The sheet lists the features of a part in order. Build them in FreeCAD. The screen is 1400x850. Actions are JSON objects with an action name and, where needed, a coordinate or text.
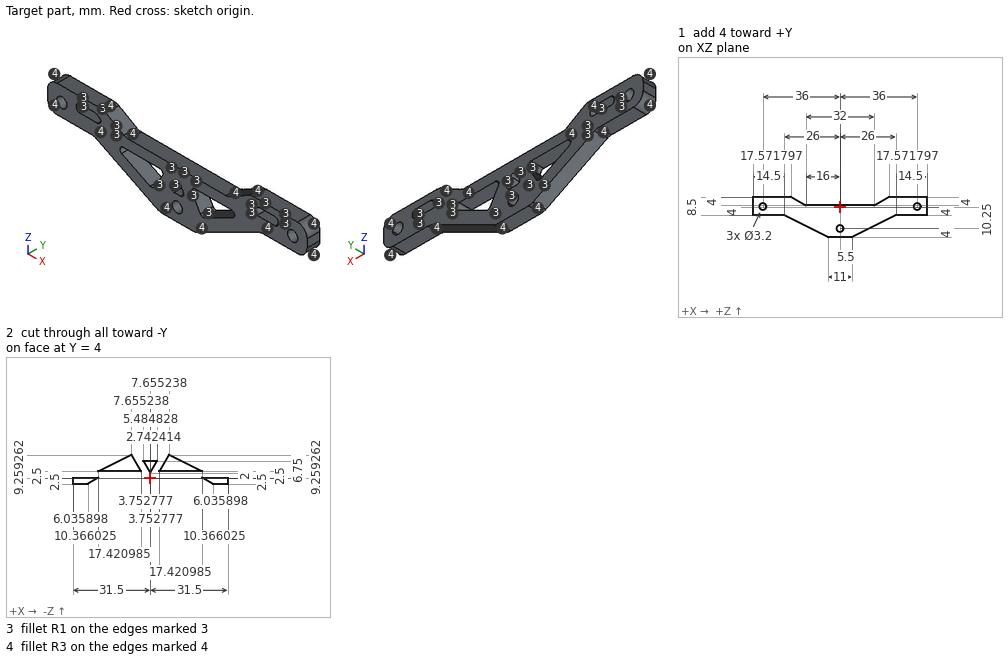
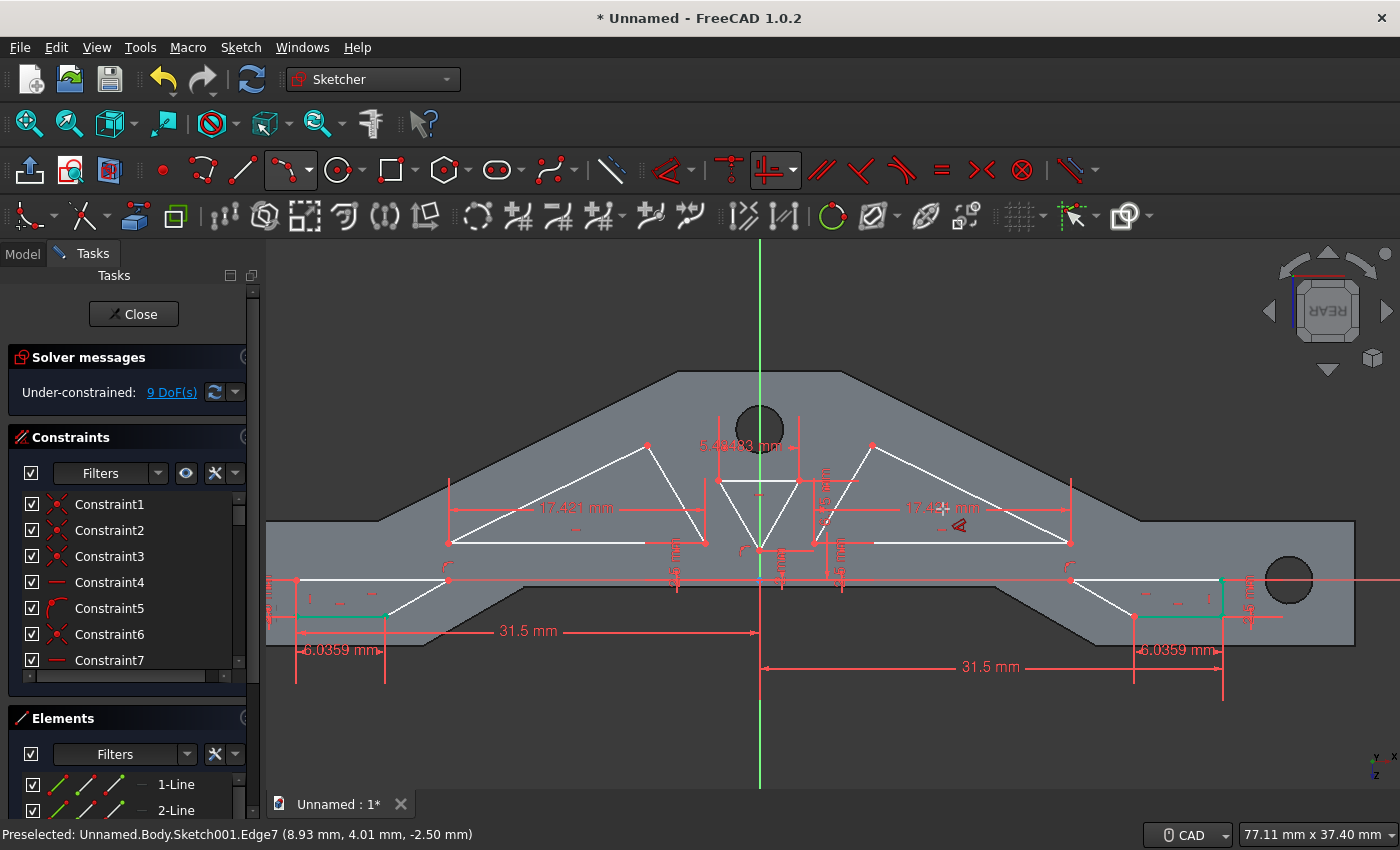
{"action": "left_click", "coordinate": [403, 580]}
{"action": "left_click", "coordinate": [426, 614]}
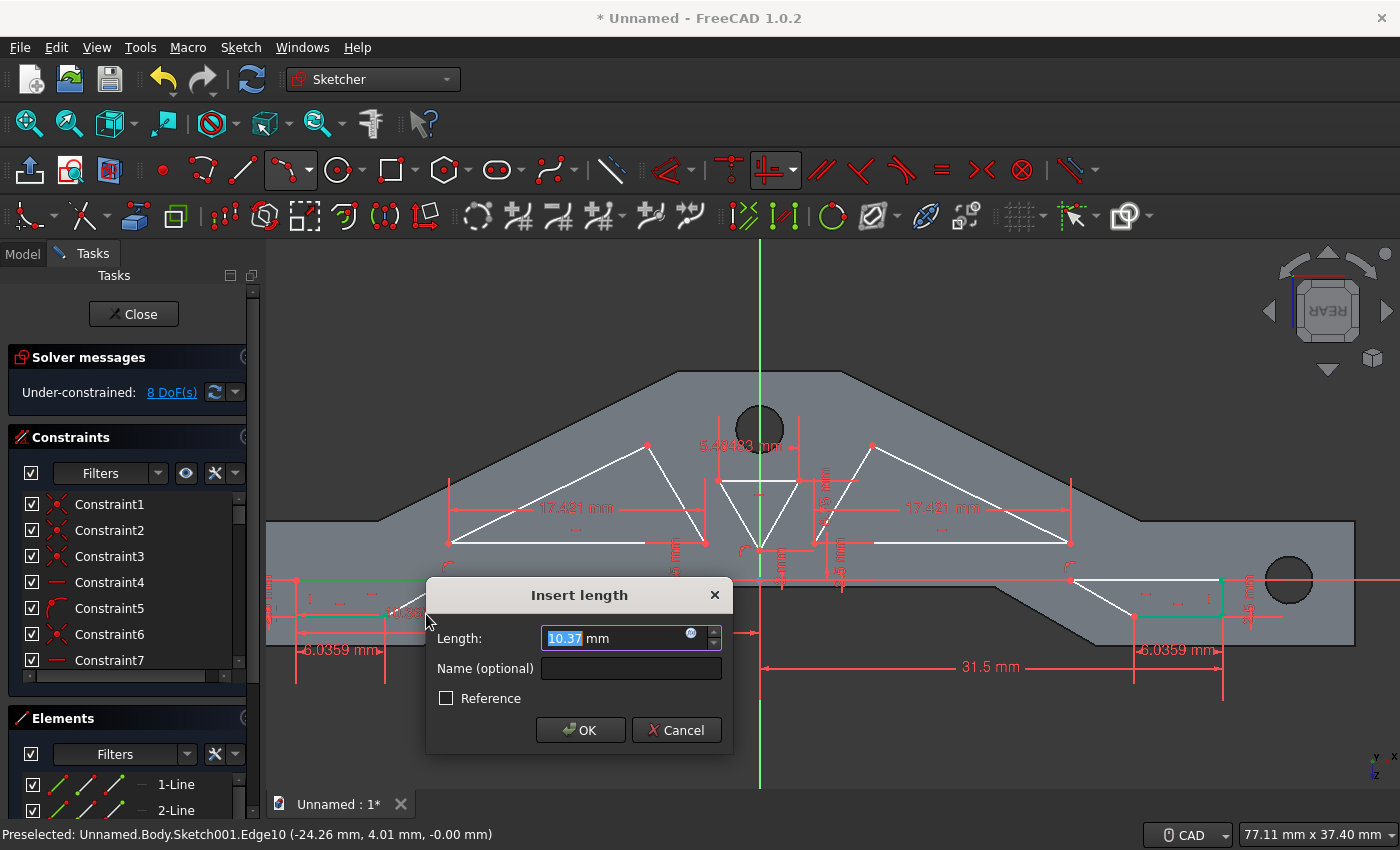
{"action": "type", "text": "10.366025"}
{"action": "key", "text": "Return"}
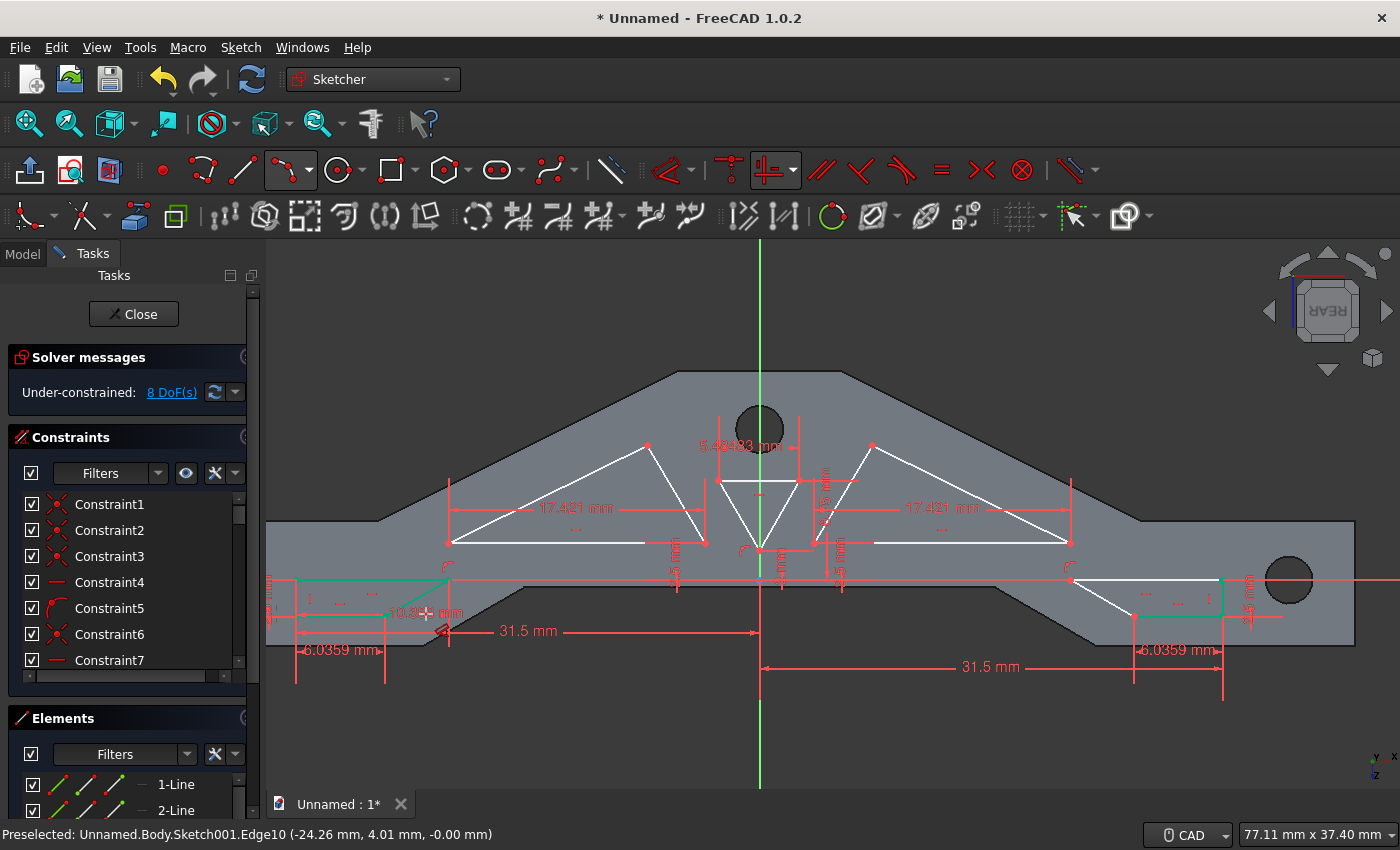
{"action": "left_click", "coordinate": [1177, 580]}
{"action": "left_click", "coordinate": [1094, 614]}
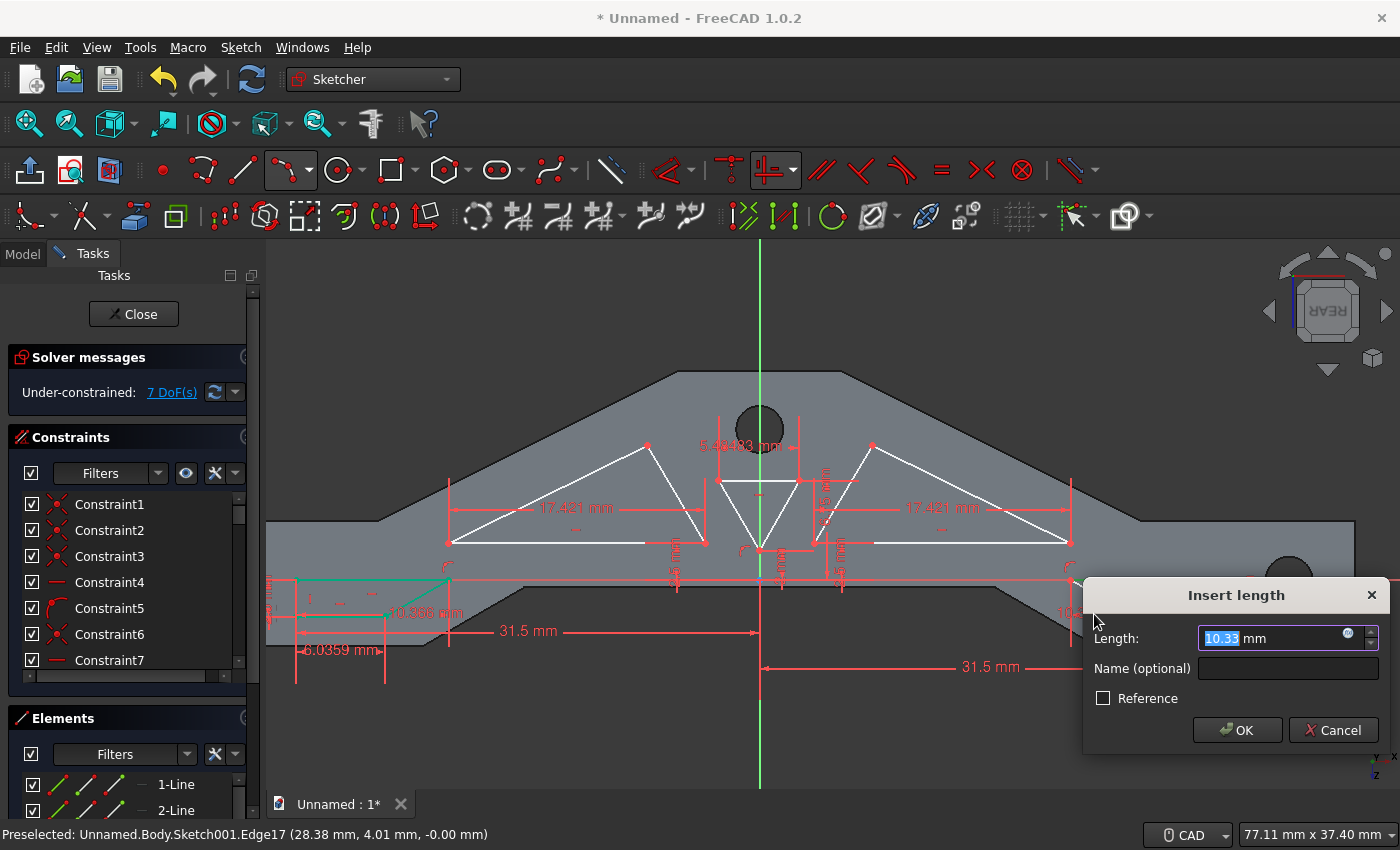
{"action": "type", "text": "10.366025"}
{"action": "key", "text": "Return"}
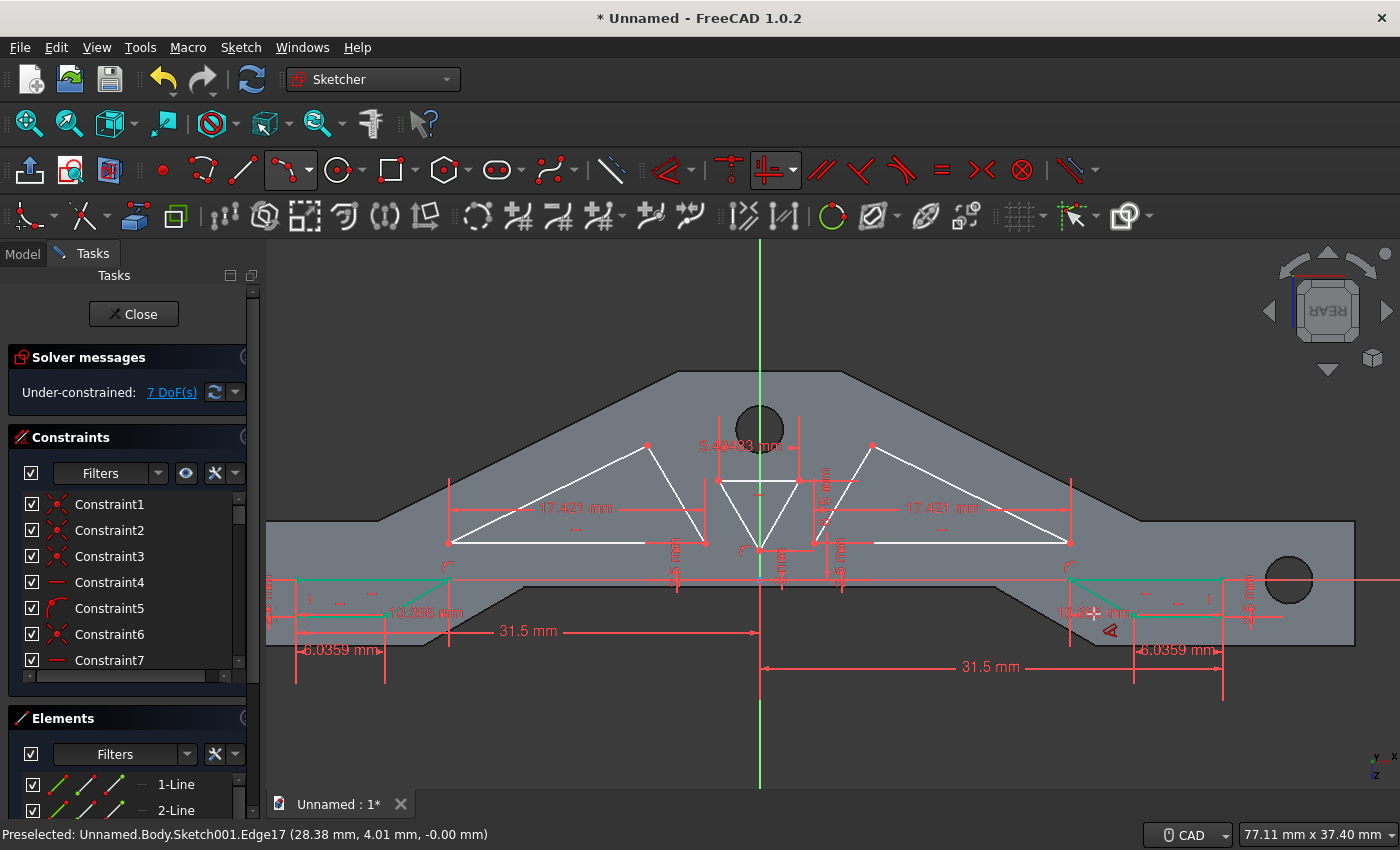
{"action": "left_click", "coordinate": [705, 543]}
{"action": "left_click", "coordinate": [732, 614]}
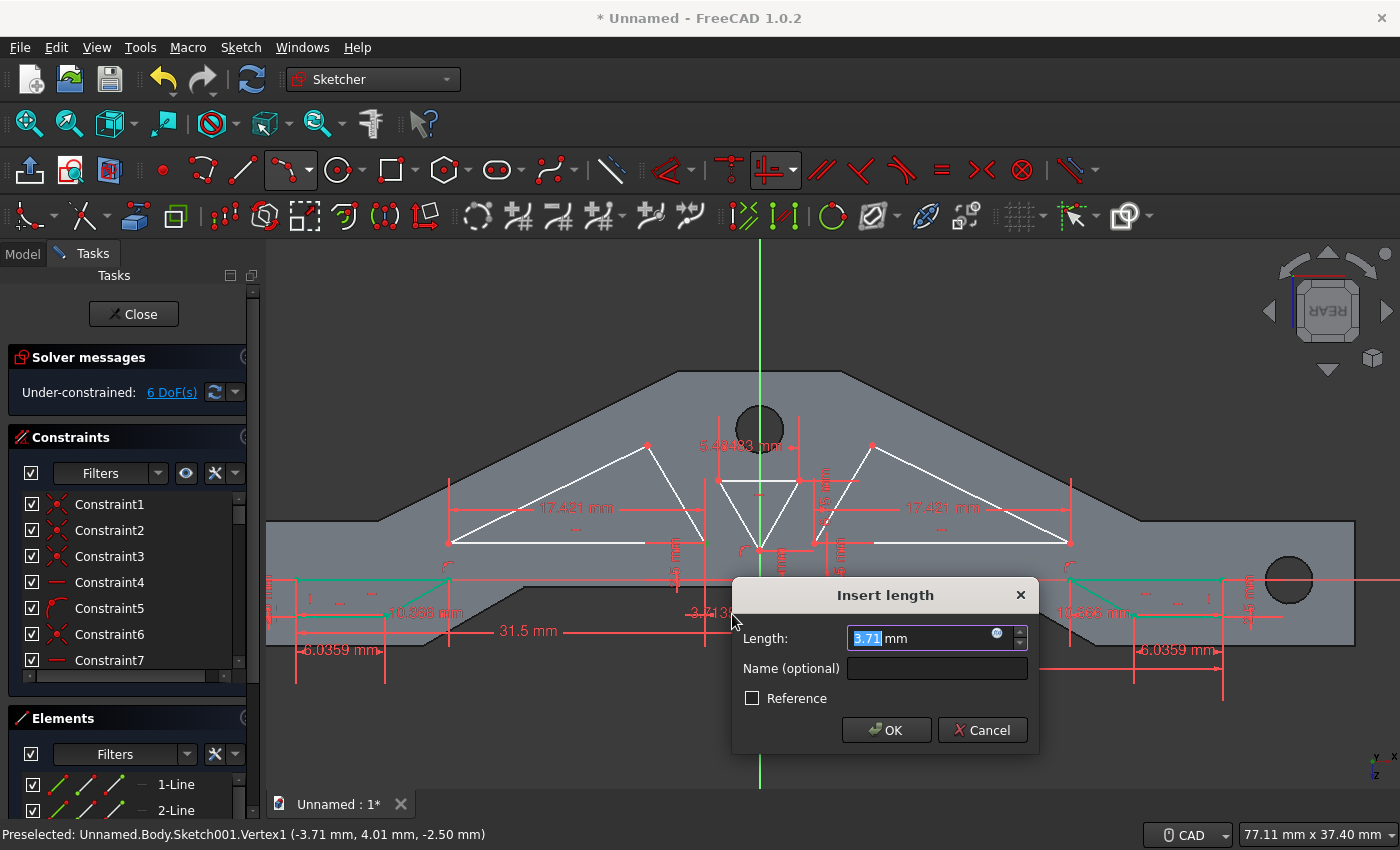
{"action": "type", "text": "3.752777"}
{"action": "key", "text": "Return"}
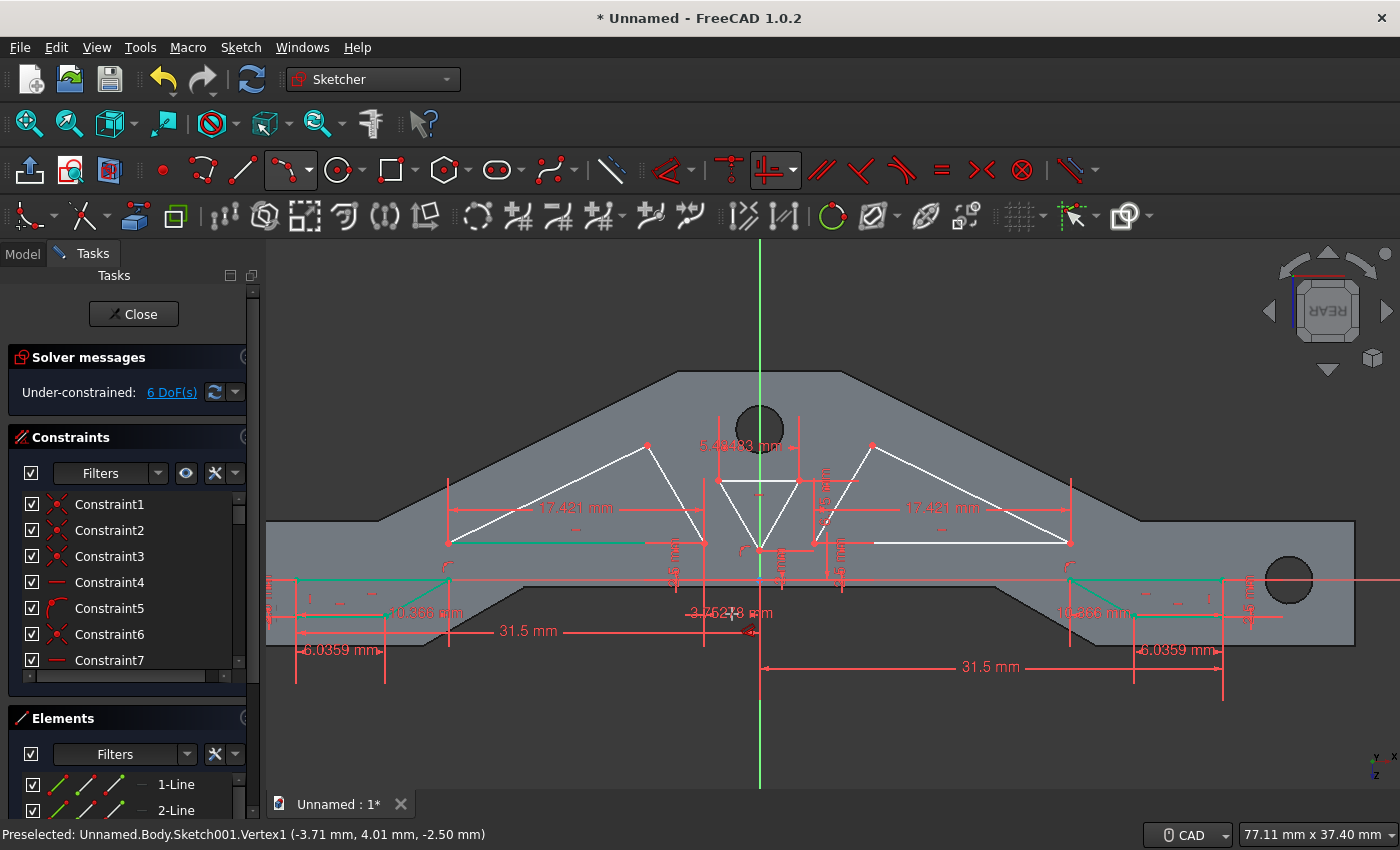
{"action": "left_click", "coordinate": [647, 446]}
{"action": "left_click", "coordinate": [703, 412]}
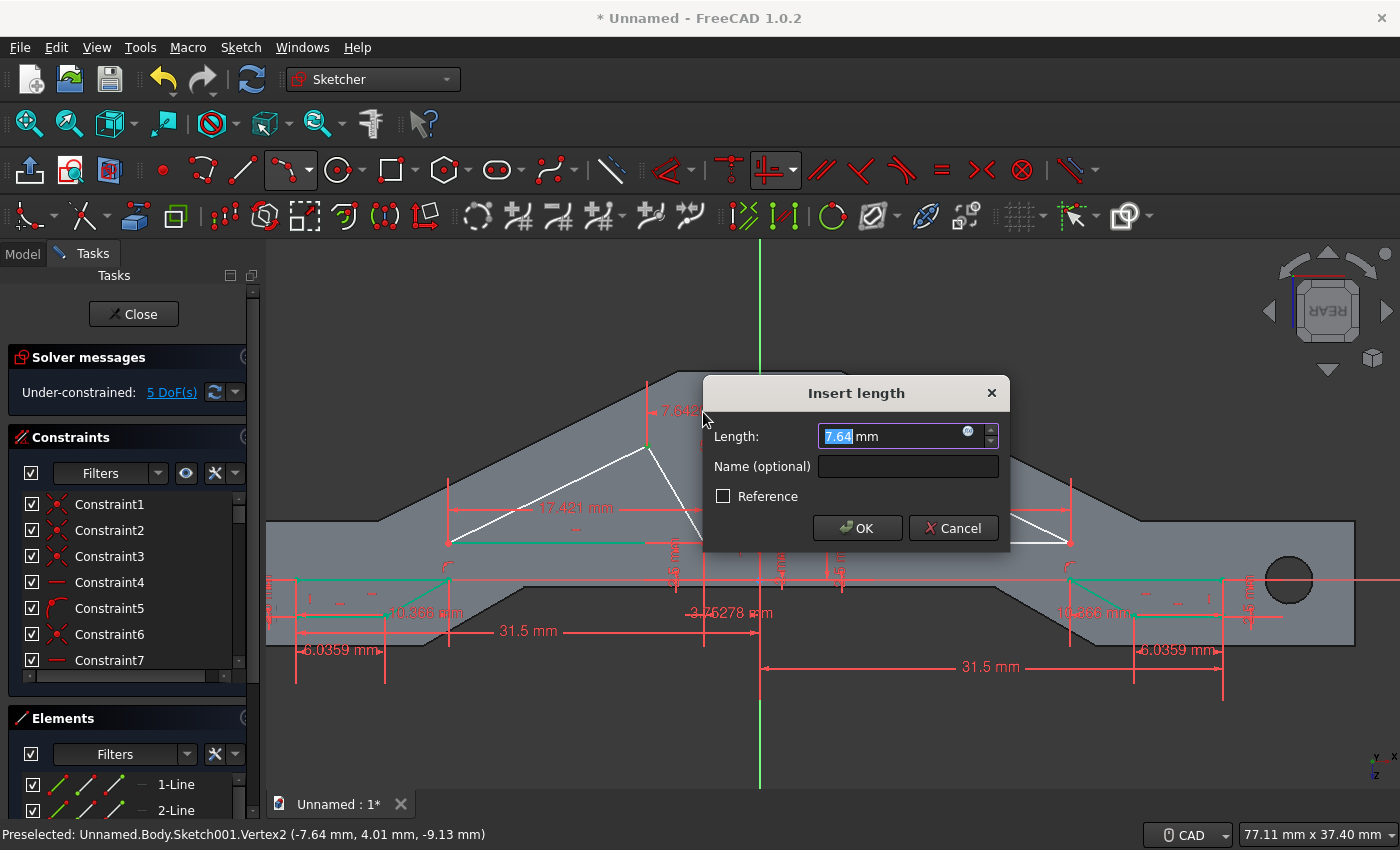
{"action": "type", "text": "7.655238"}
{"action": "key", "text": "Return"}